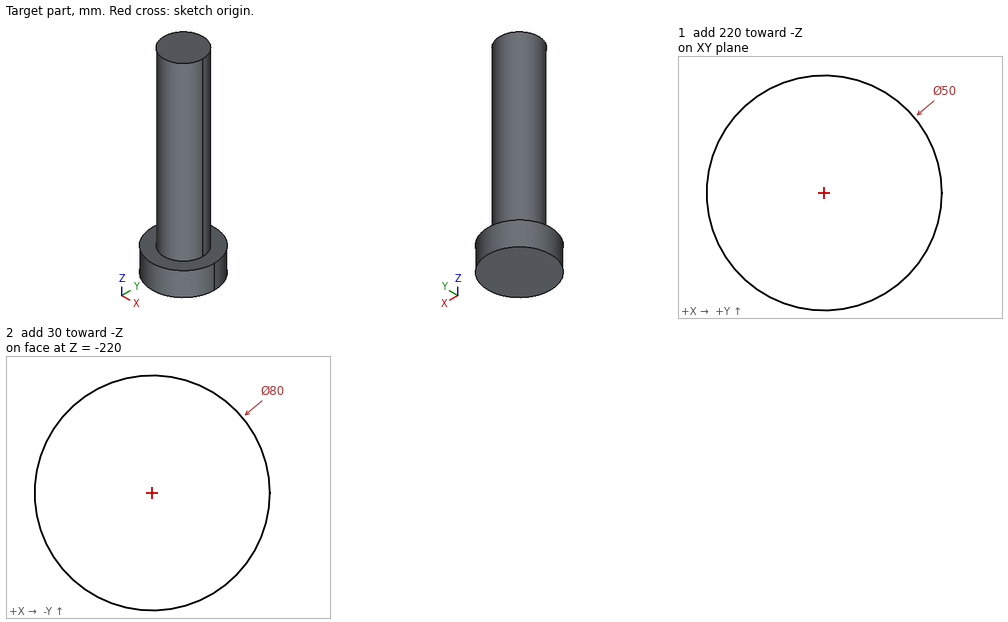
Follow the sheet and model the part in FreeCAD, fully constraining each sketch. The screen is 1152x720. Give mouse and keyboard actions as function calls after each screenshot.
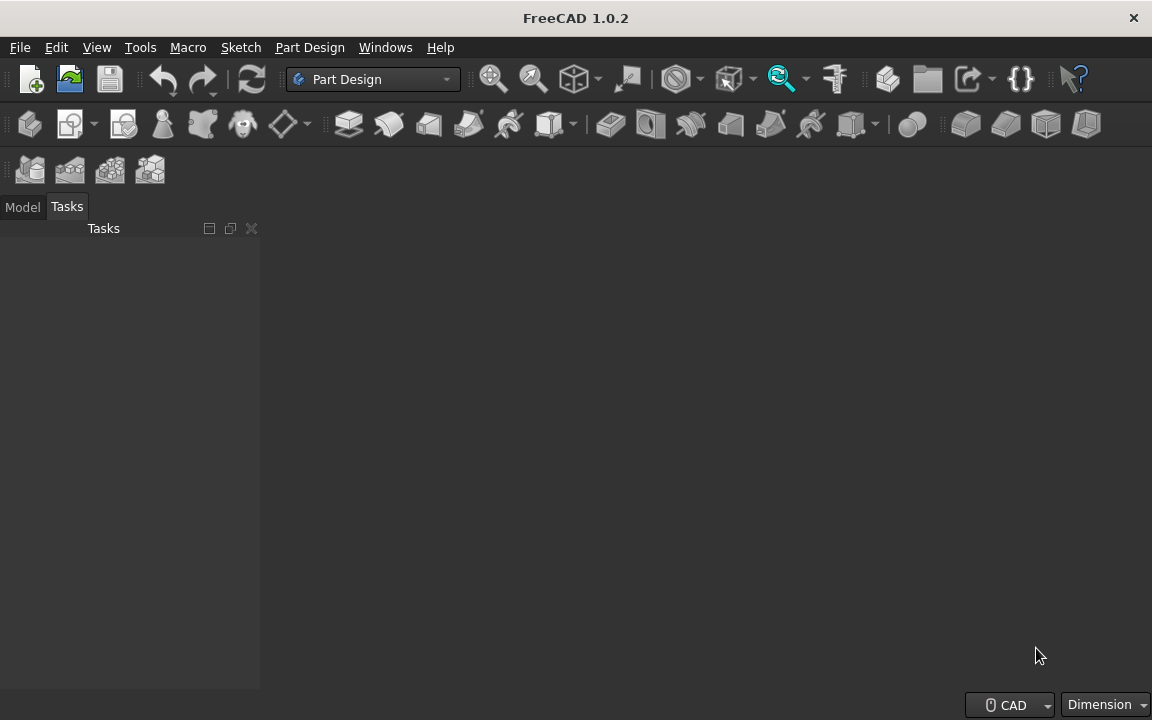
click(30, 80)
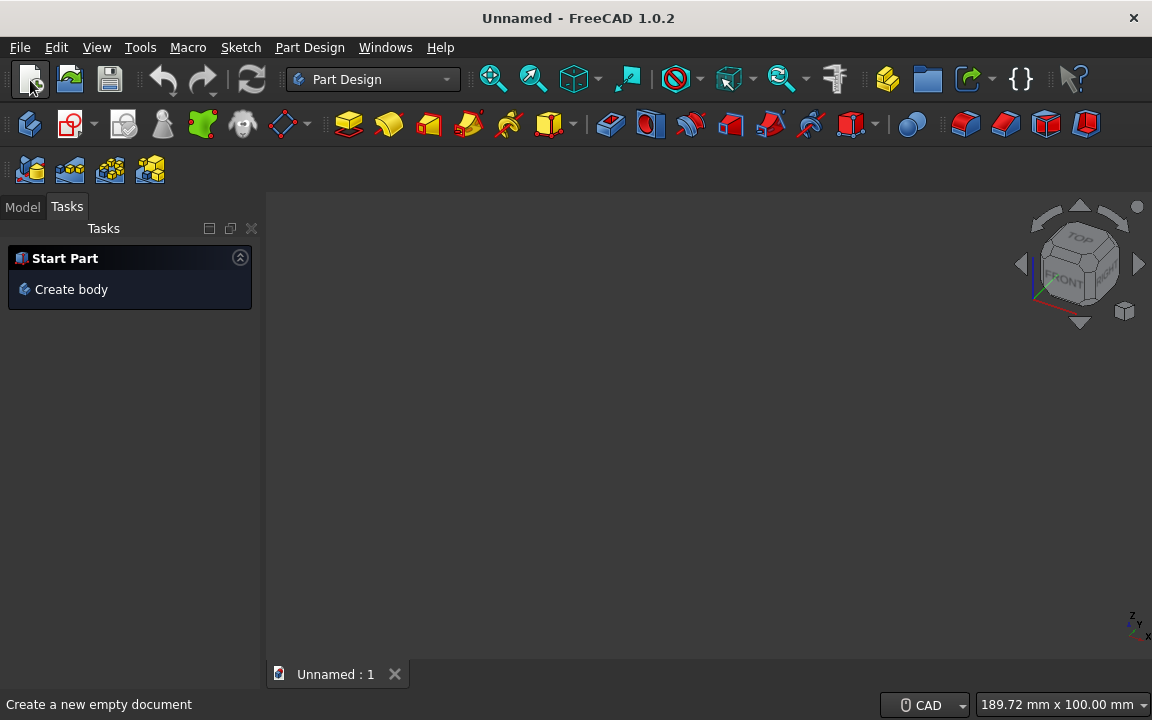
click(70, 124)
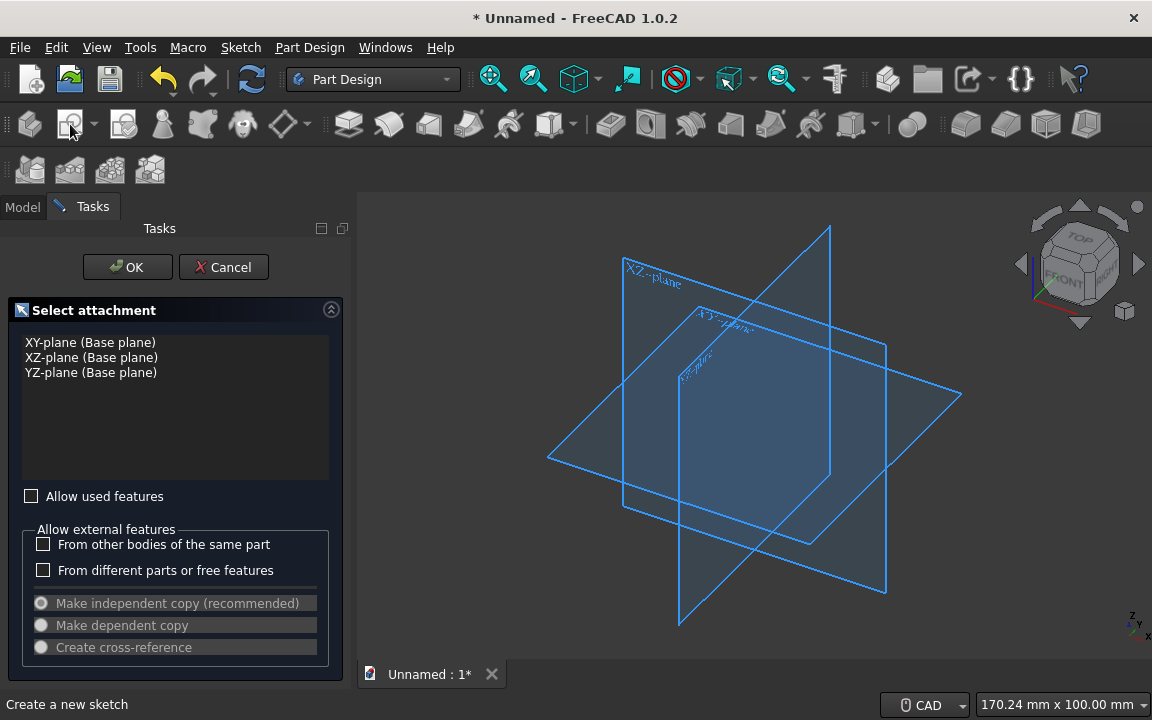
click(82, 342)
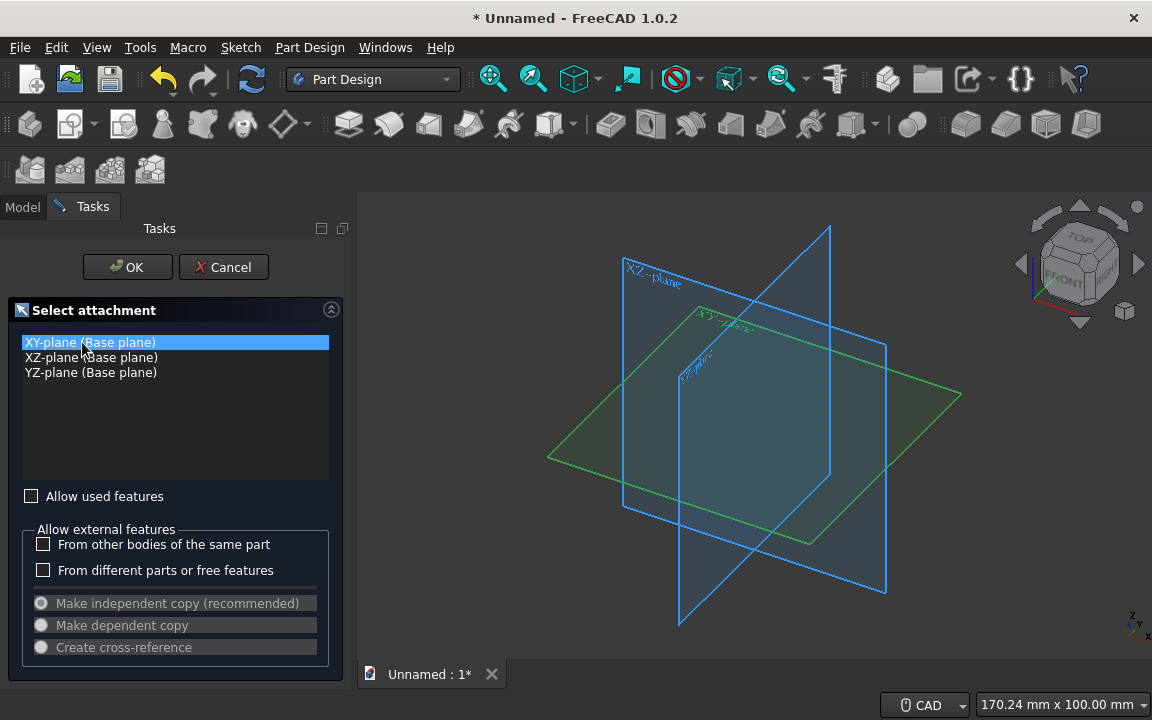
click(128, 267)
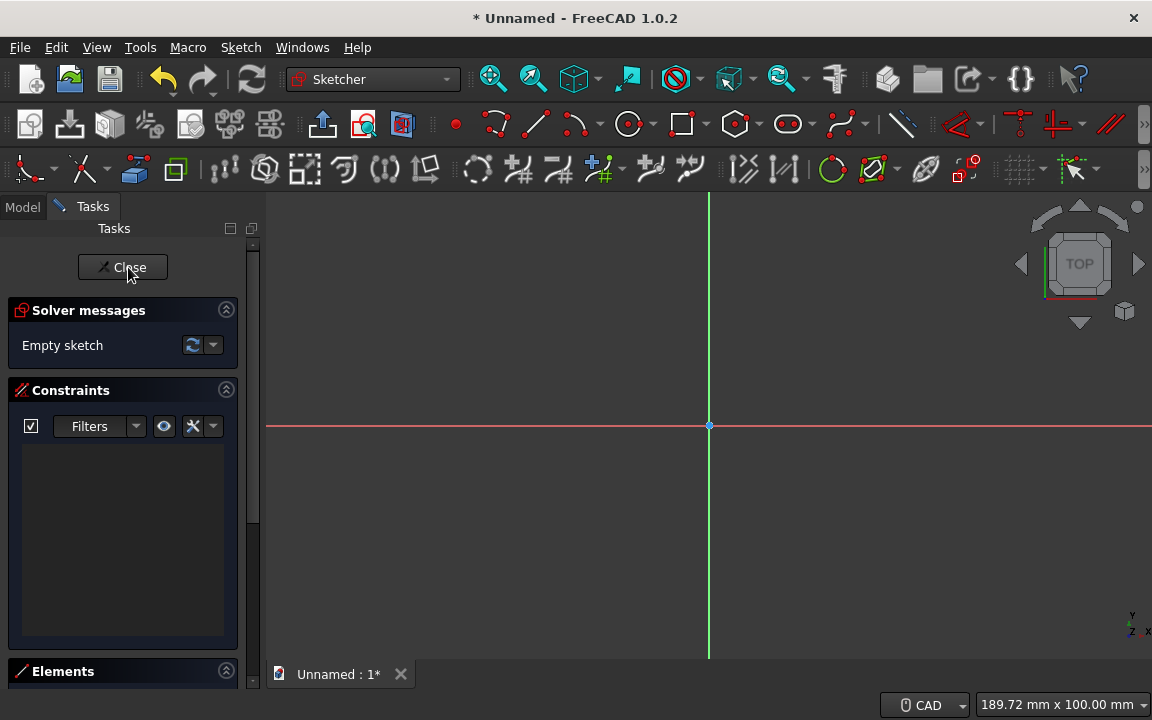
click(630, 124)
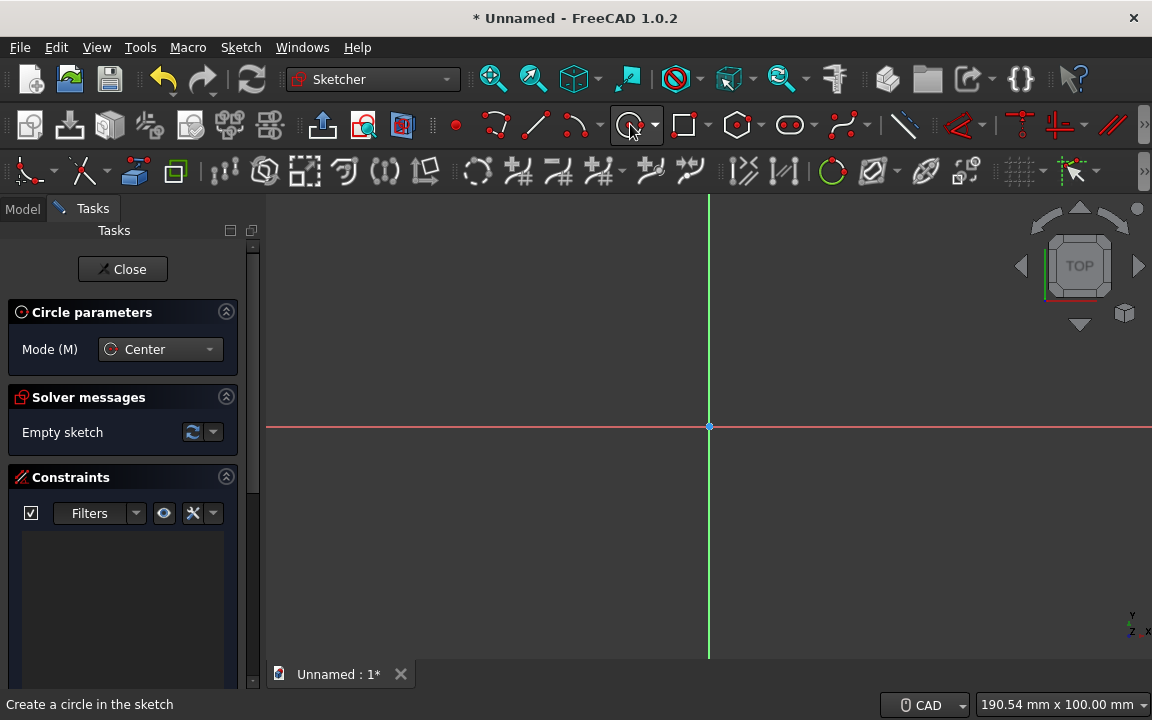
click(709, 426)
move(791, 344)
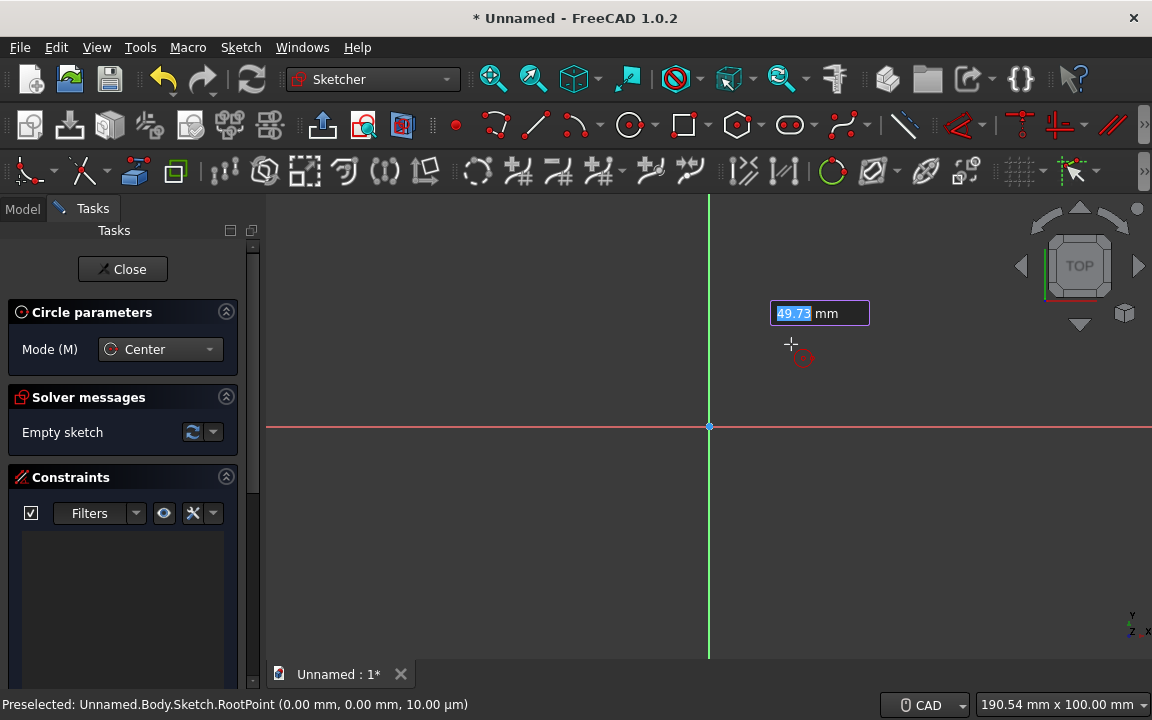
text(50)
key(Return)
key(Escape)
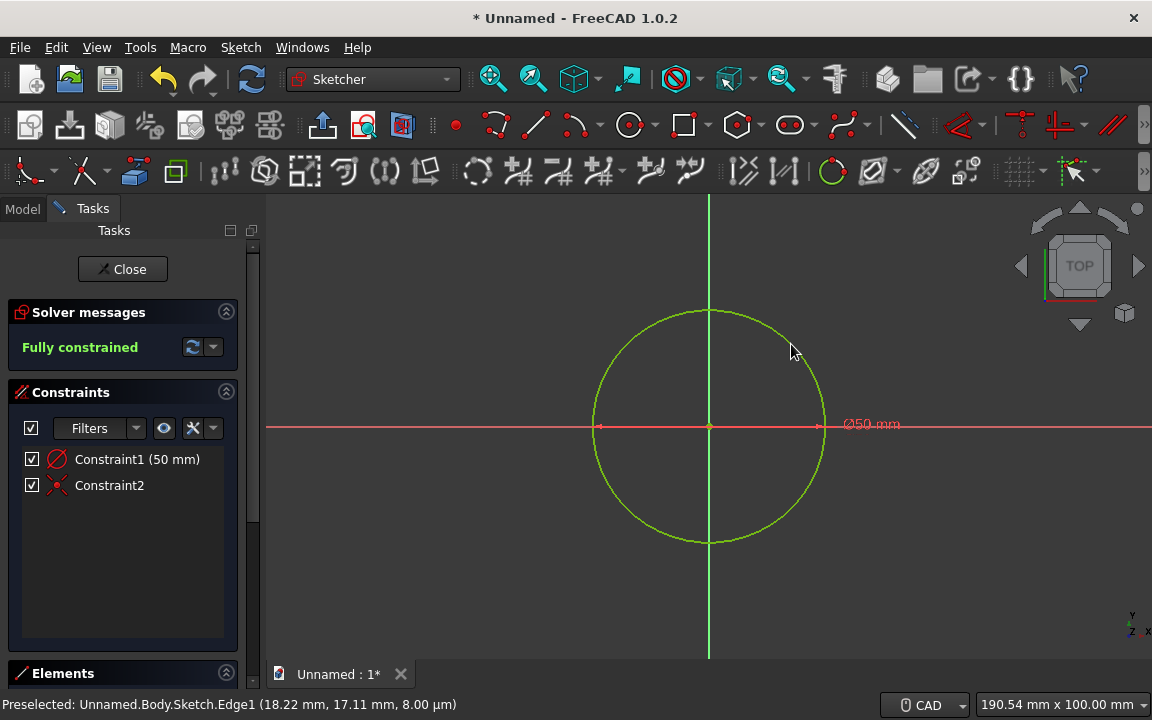
click(123, 269)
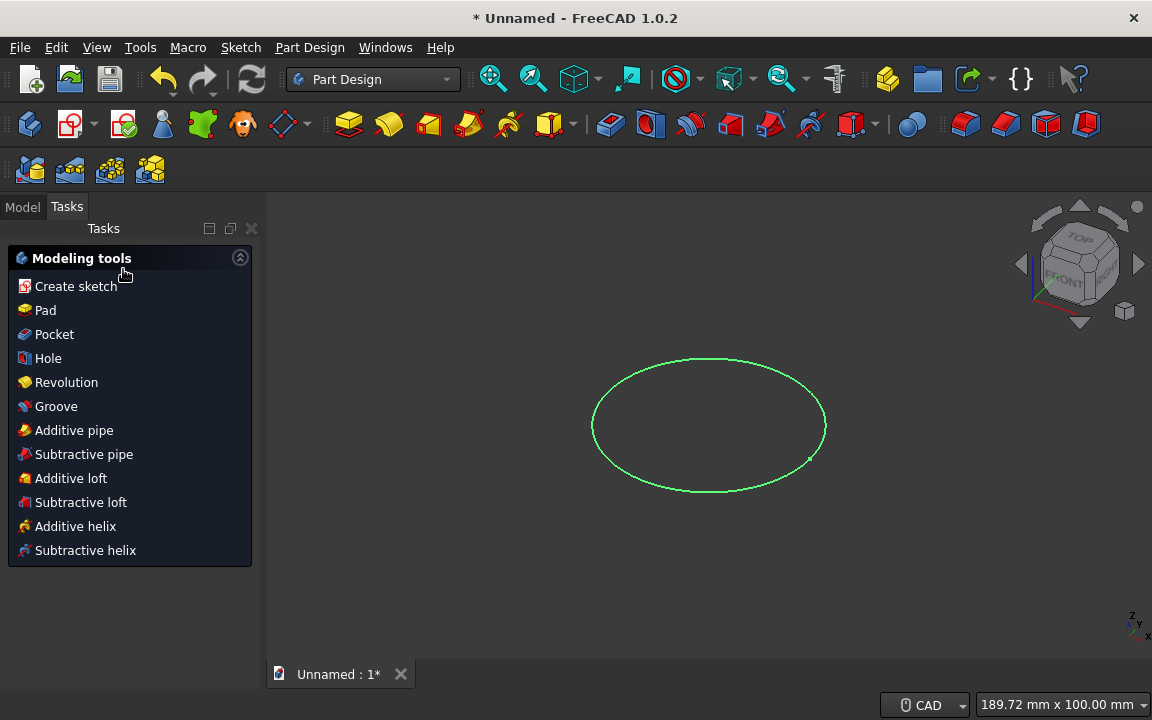
click(350, 124)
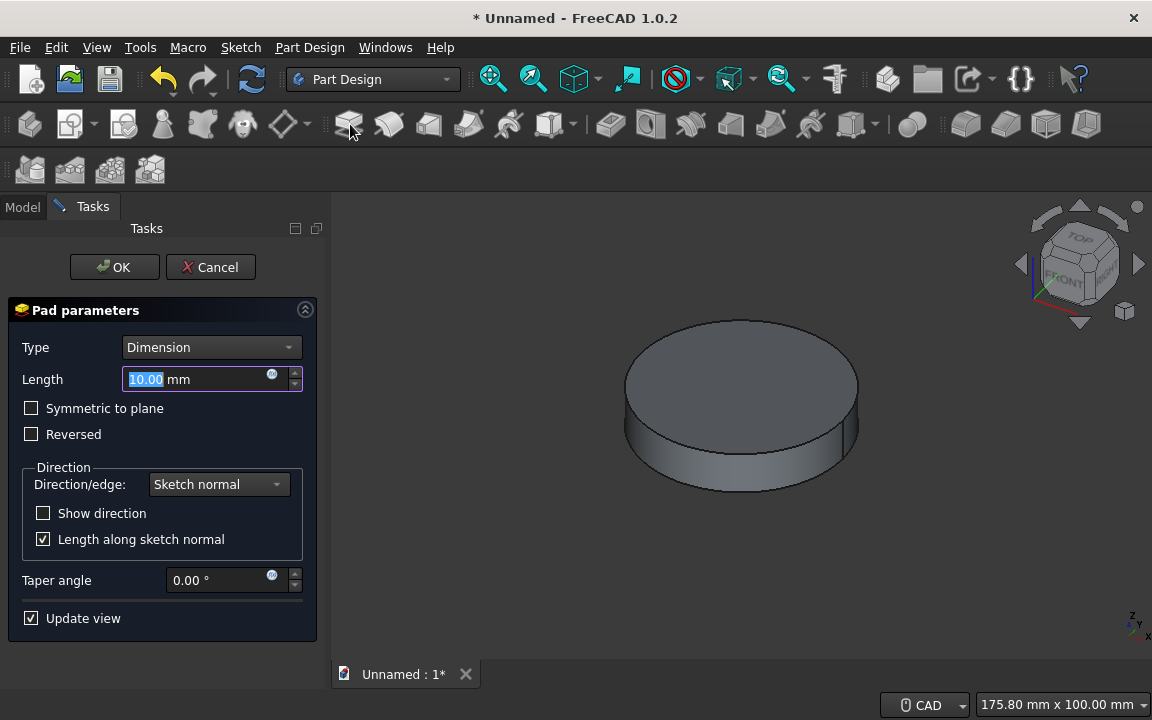
text(220)
key(Tab)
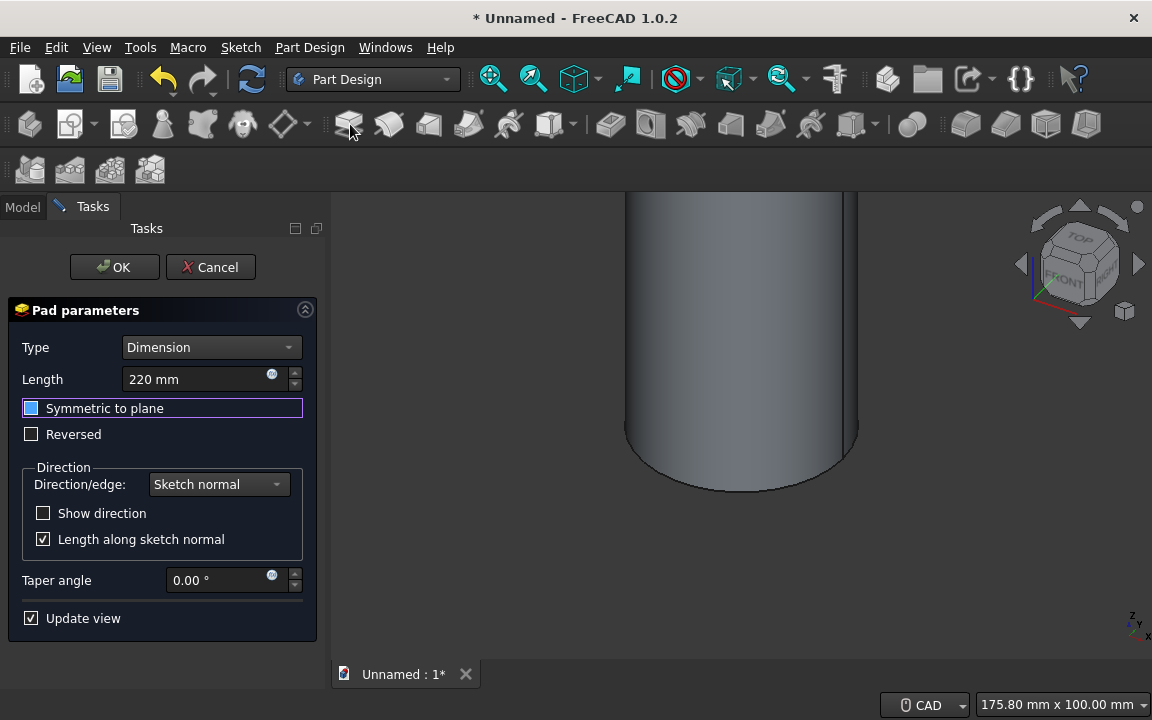
click(30, 434)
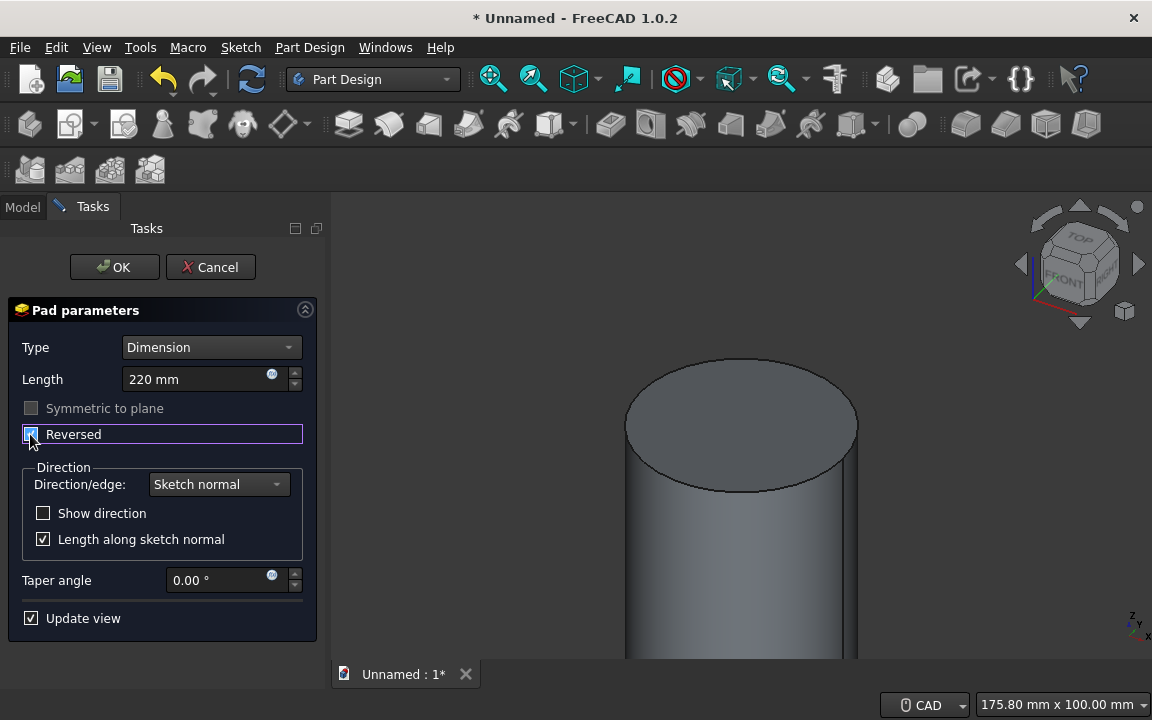
click(115, 267)